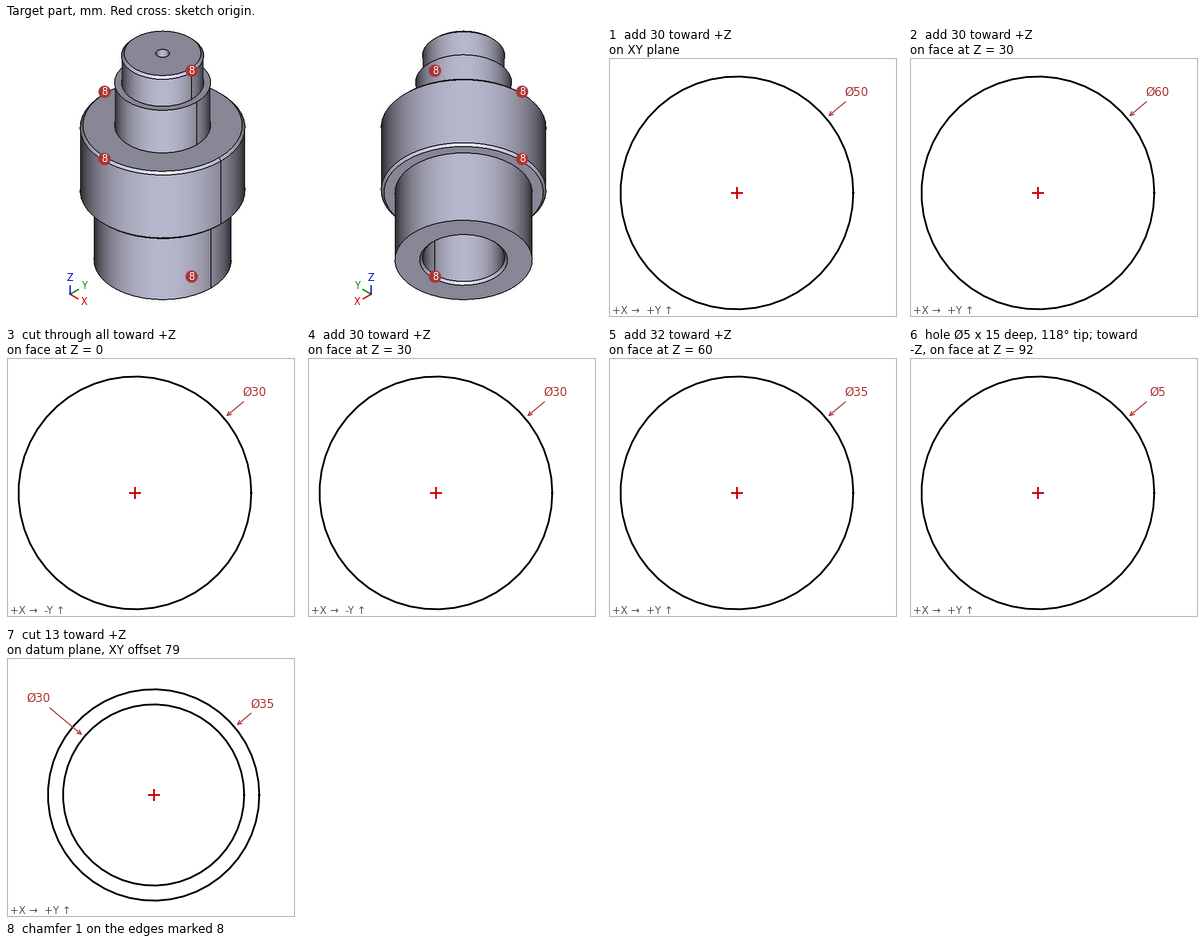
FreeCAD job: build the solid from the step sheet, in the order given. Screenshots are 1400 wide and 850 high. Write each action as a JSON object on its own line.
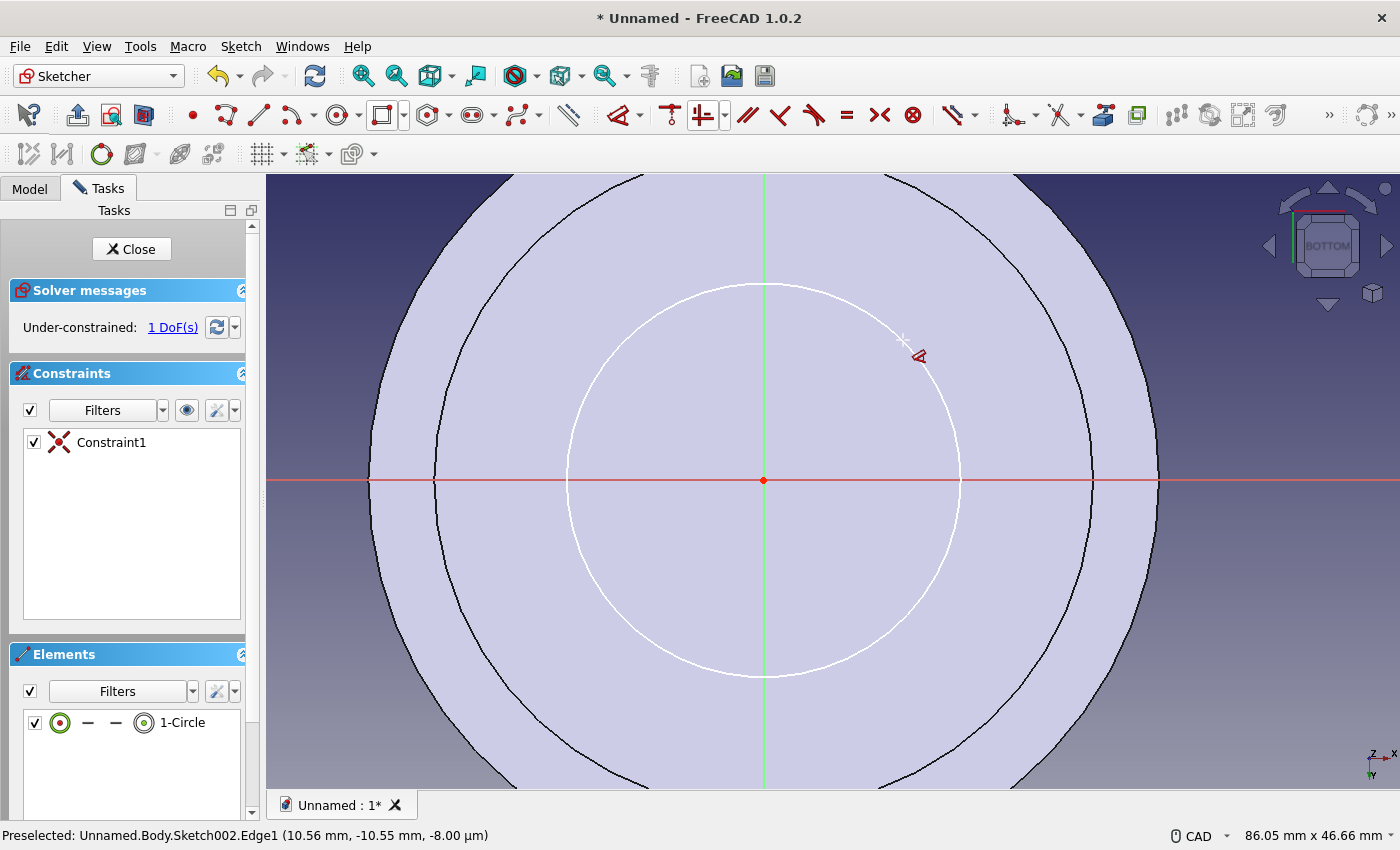
{"action": "left_click", "coordinate": [903, 341]}
{"action": "left_click", "coordinate": [926, 318]}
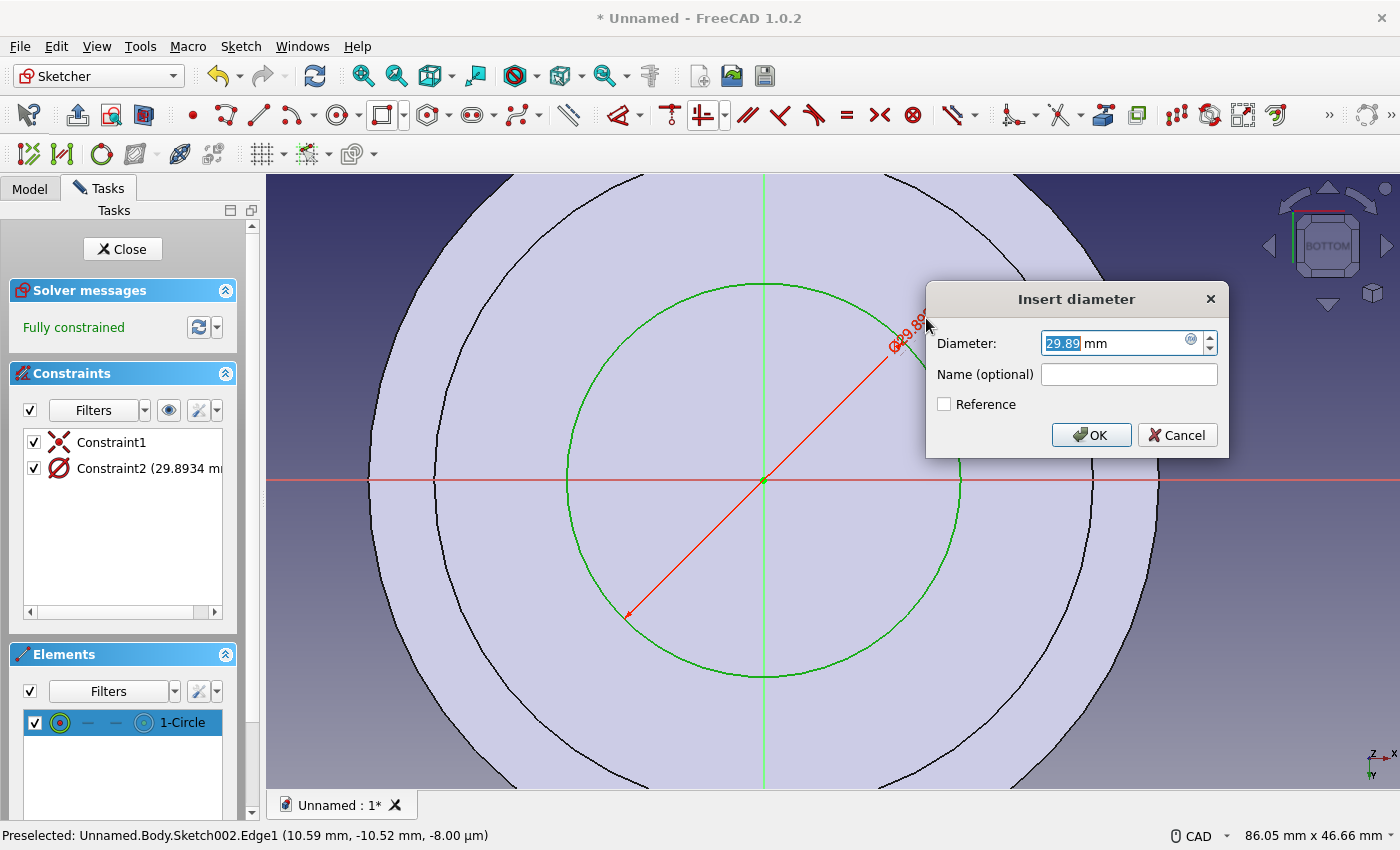
{"action": "type", "text": "30"}
{"action": "key", "text": "Return"}
{"action": "key", "text": "Escape"}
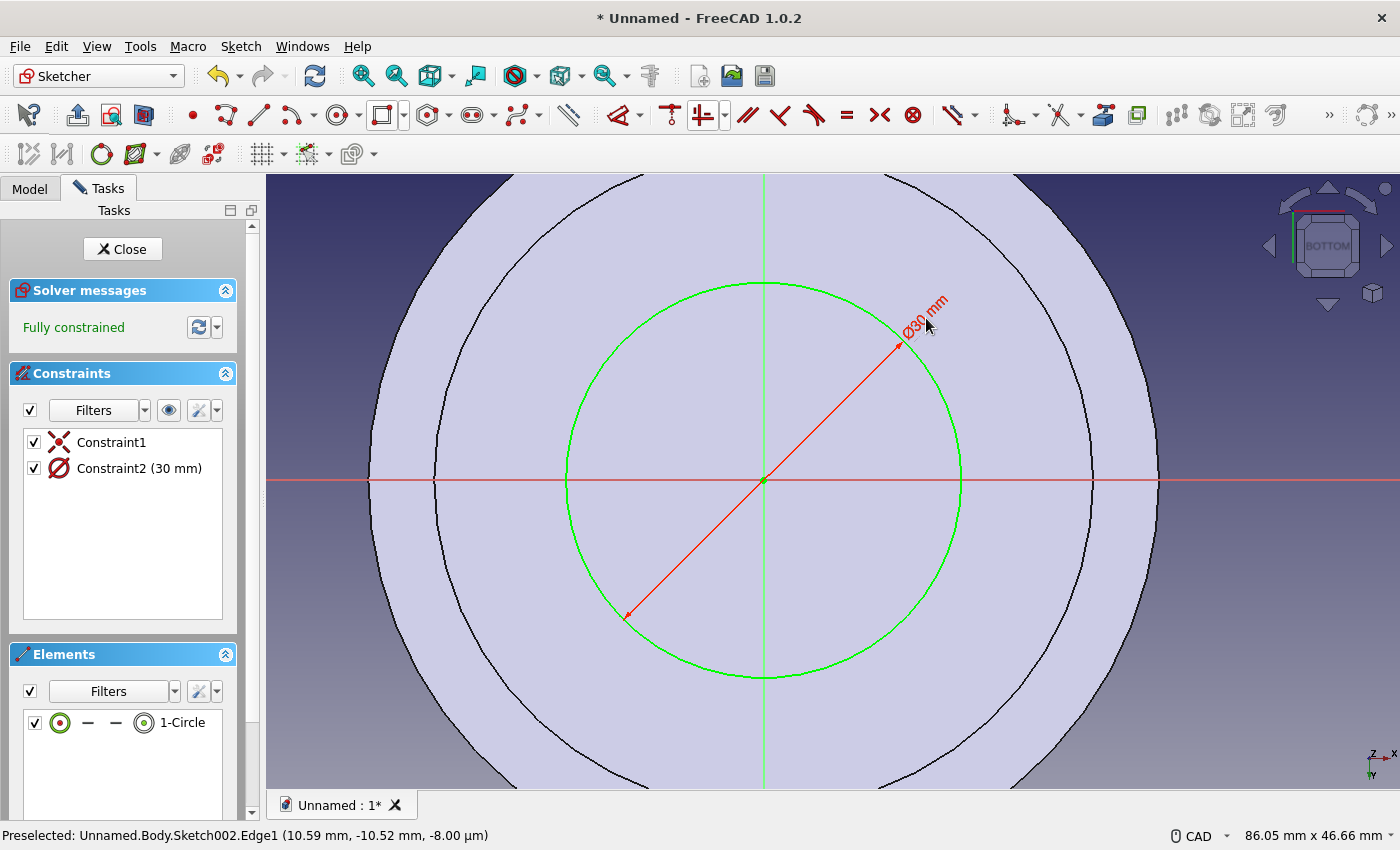
{"action": "left_click", "coordinate": [123, 249]}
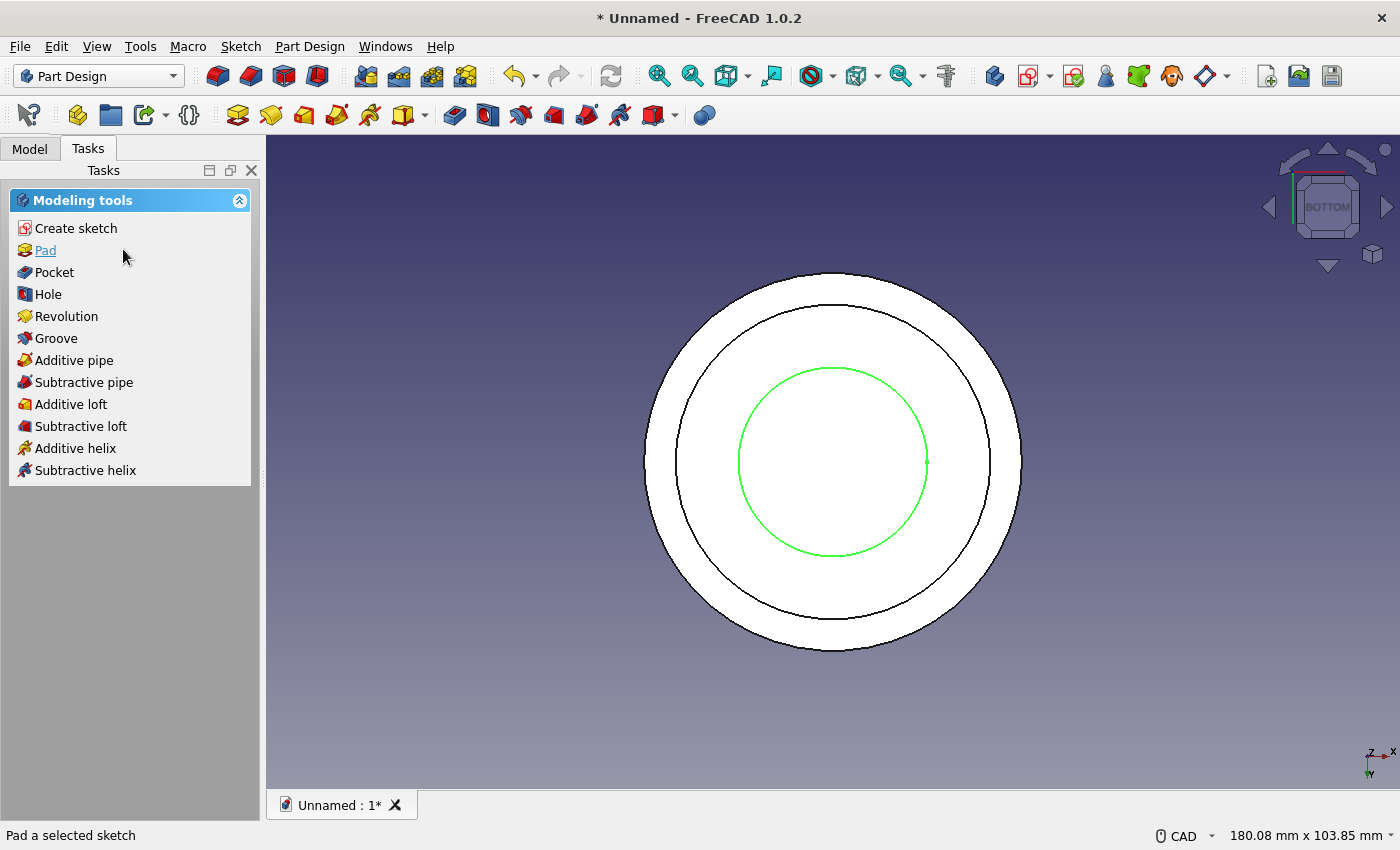
{"action": "left_click", "coordinate": [455, 116]}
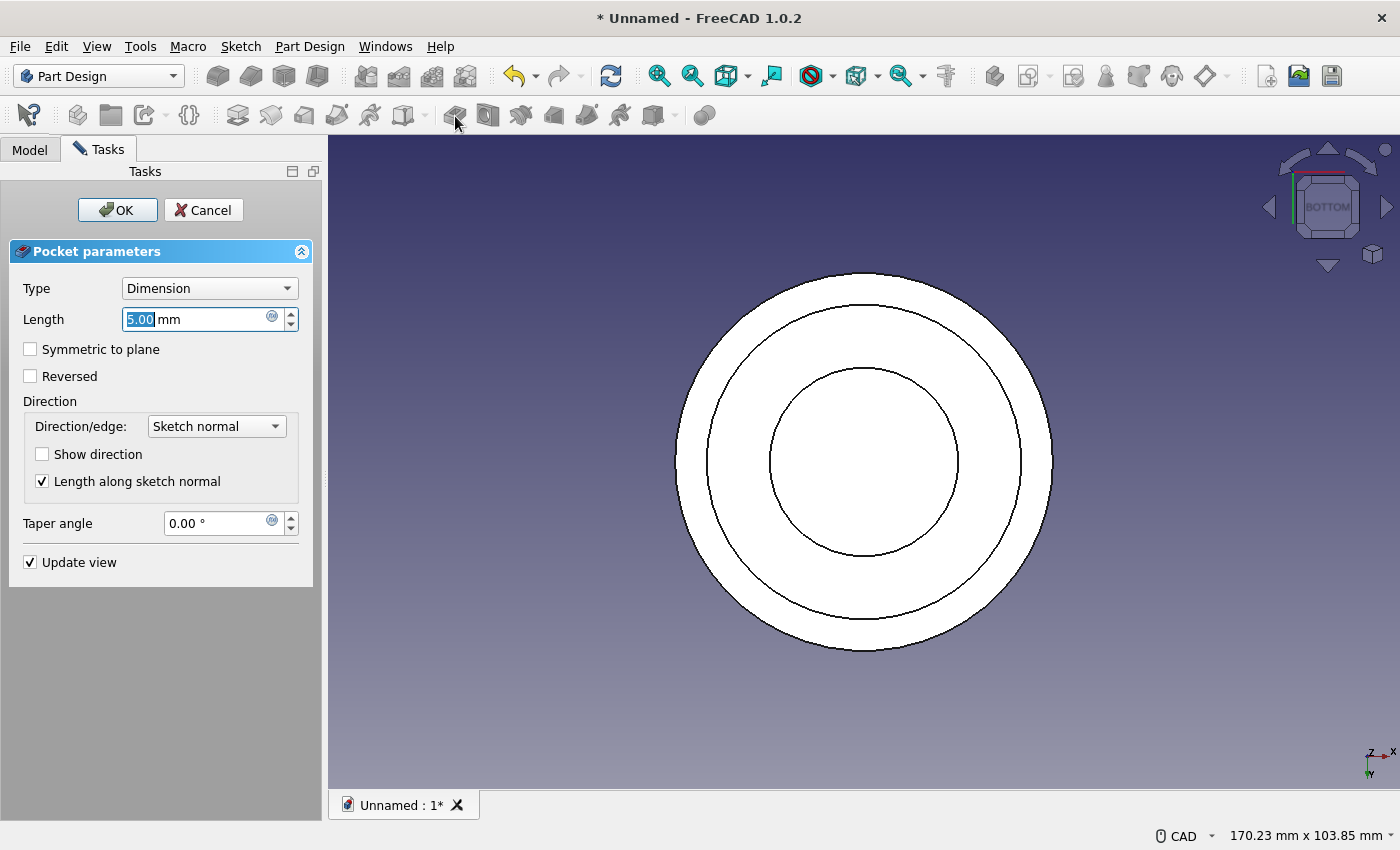
{"action": "left_click", "coordinate": [210, 288]}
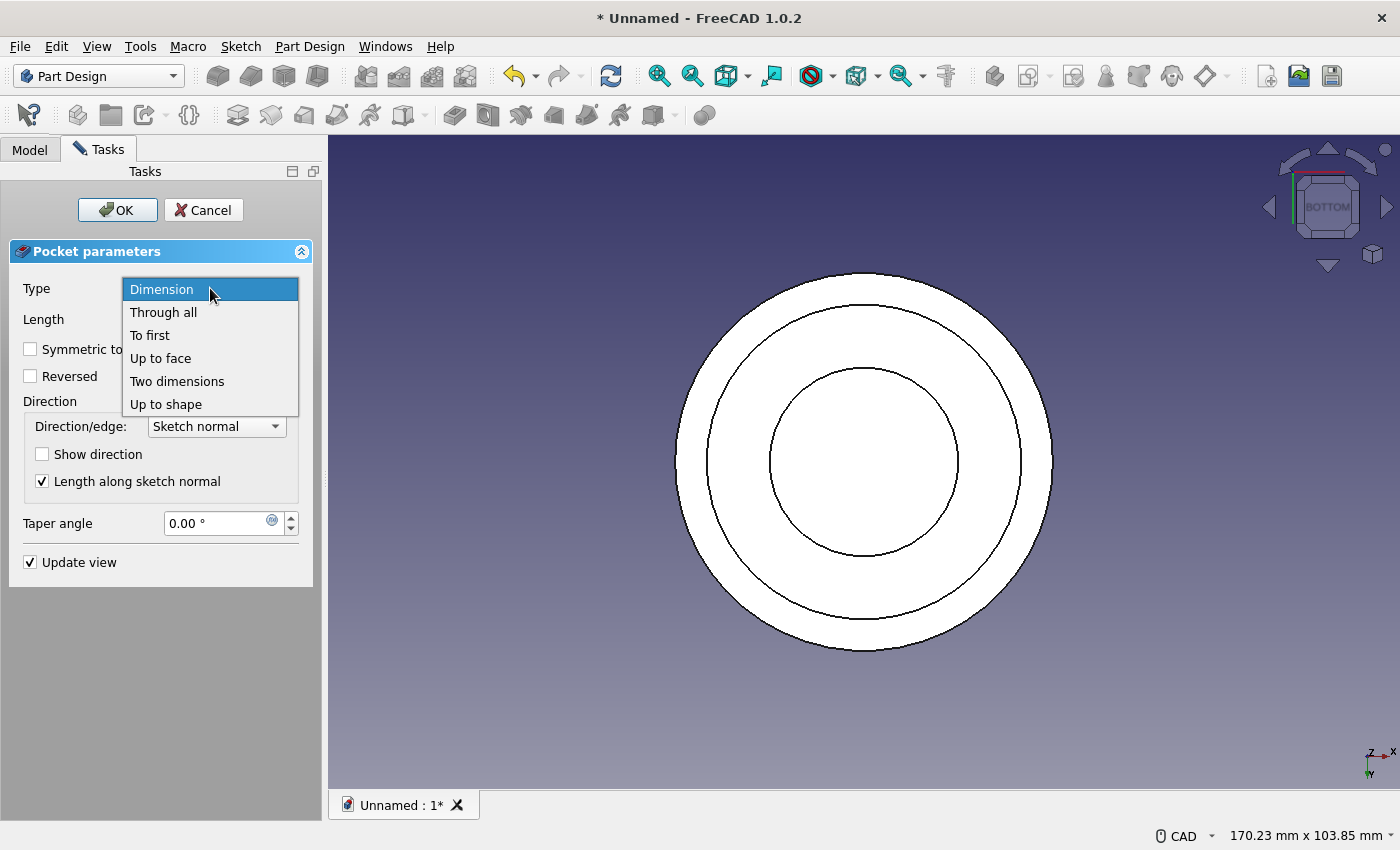
{"action": "left_click", "coordinate": [208, 312]}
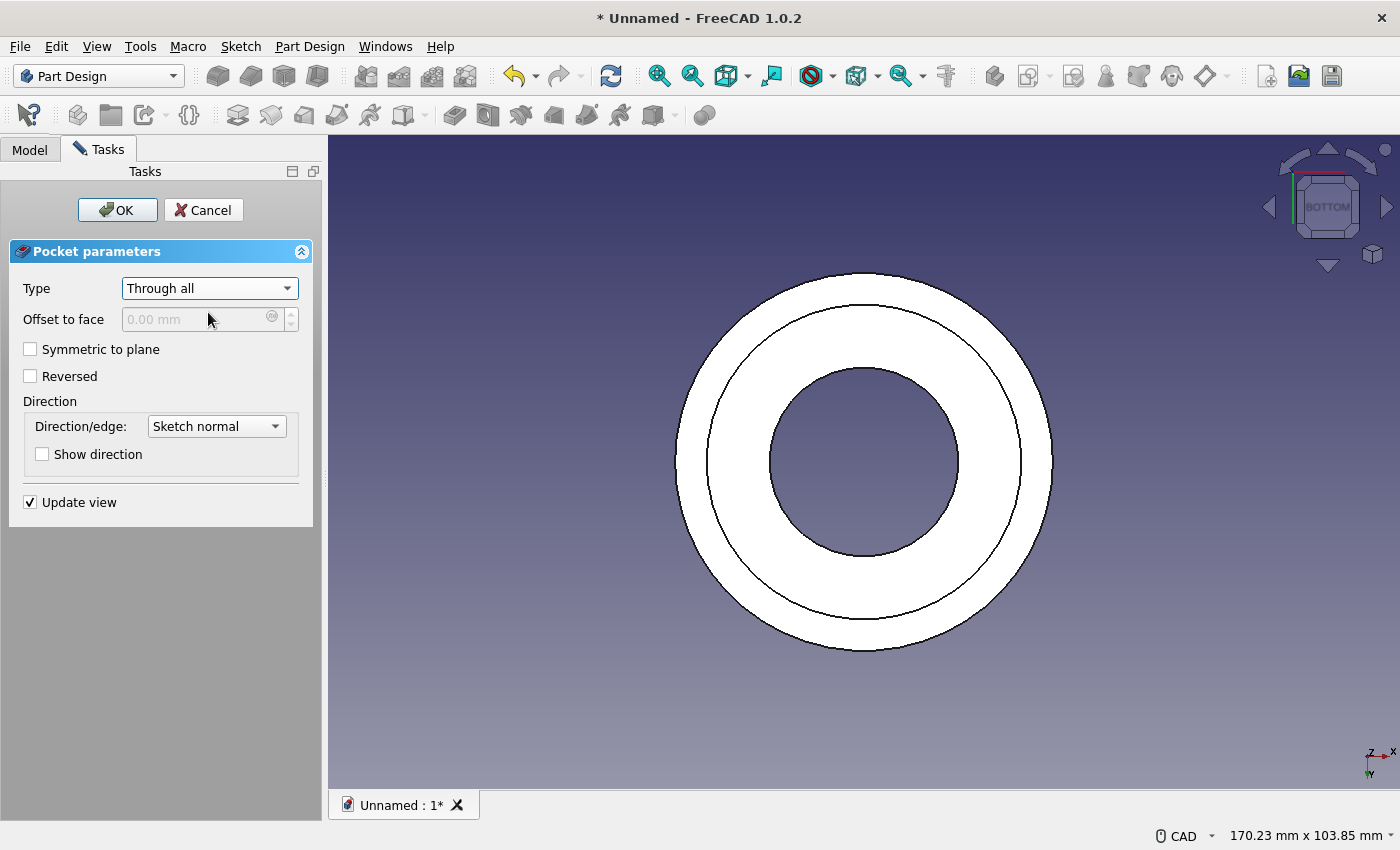
{"action": "left_click", "coordinate": [118, 210]}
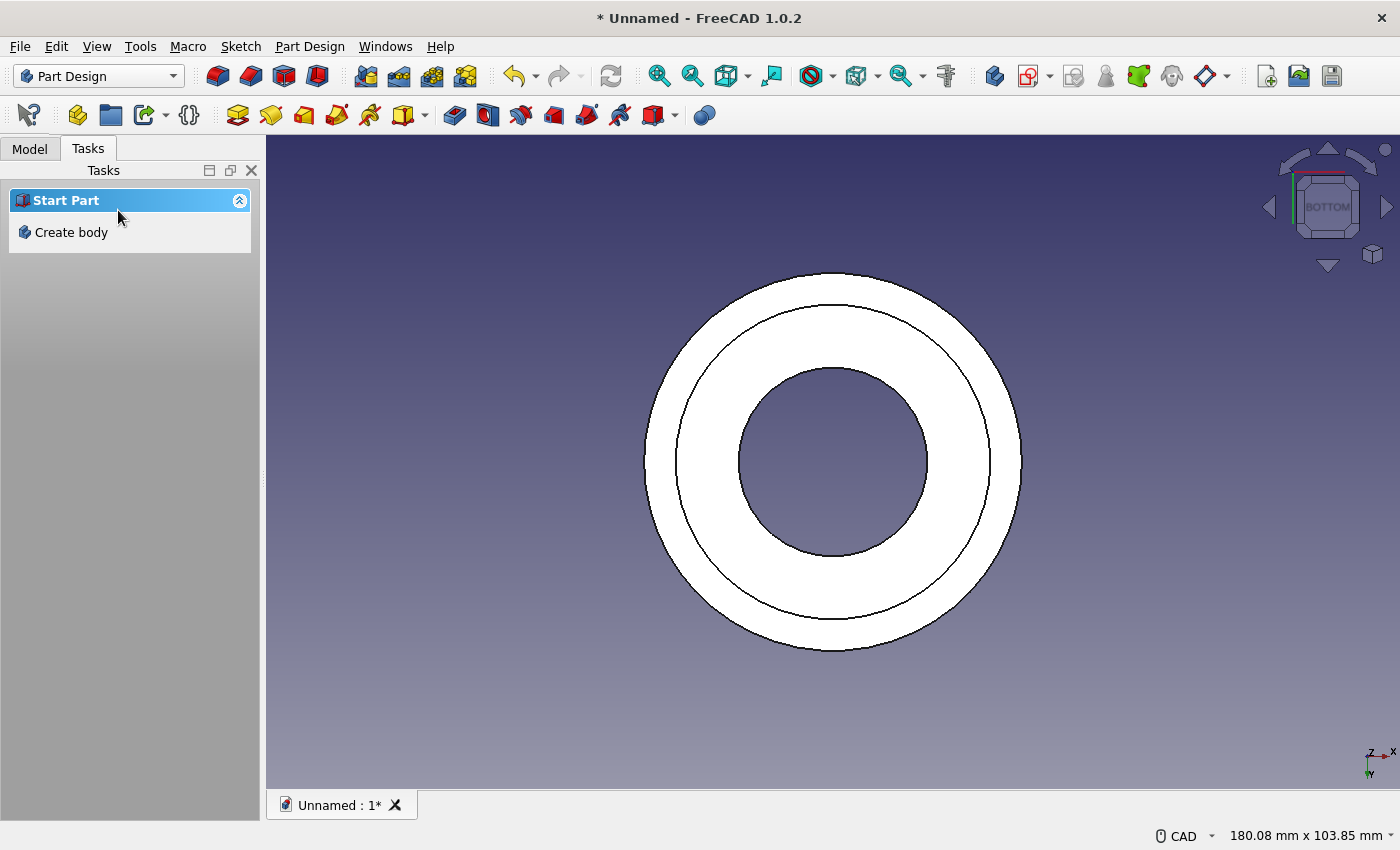
{"action": "left_click", "coordinate": [779, 623]}